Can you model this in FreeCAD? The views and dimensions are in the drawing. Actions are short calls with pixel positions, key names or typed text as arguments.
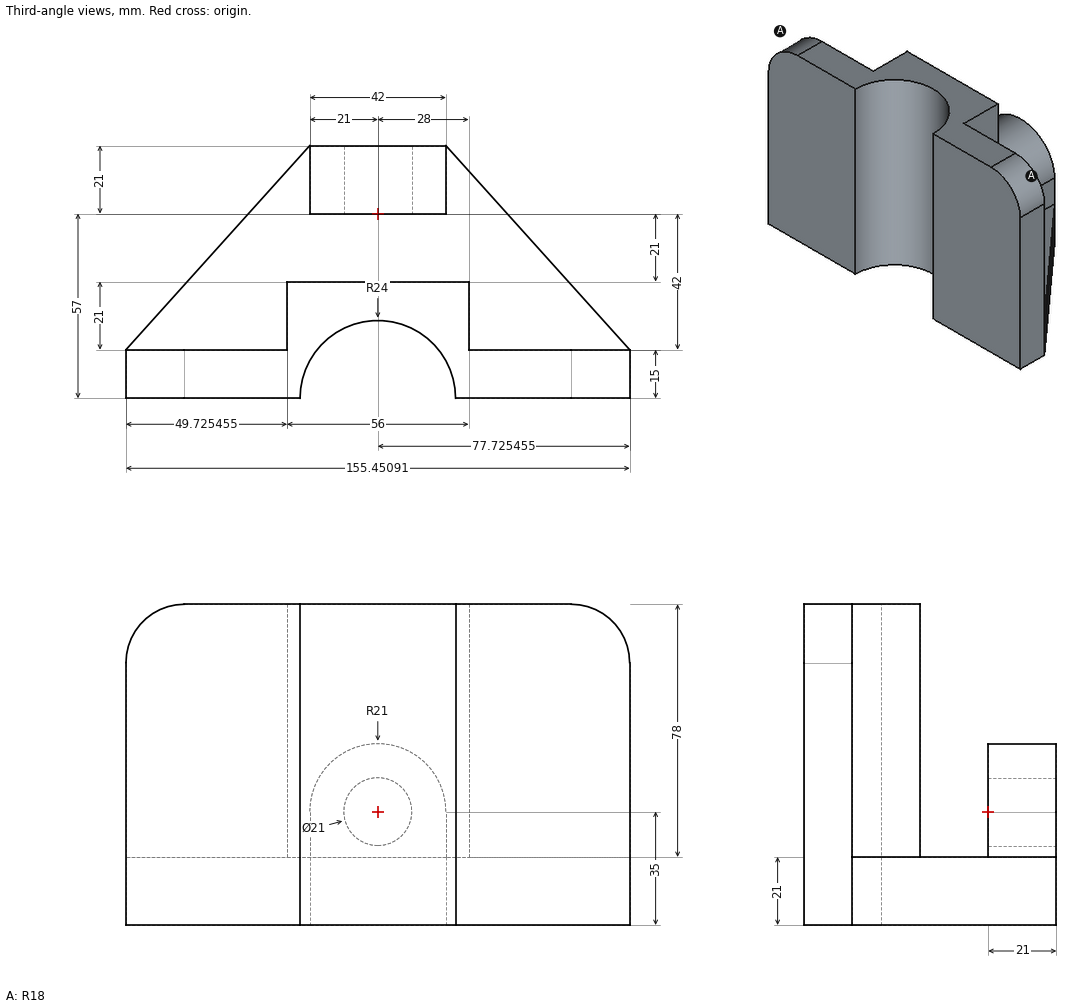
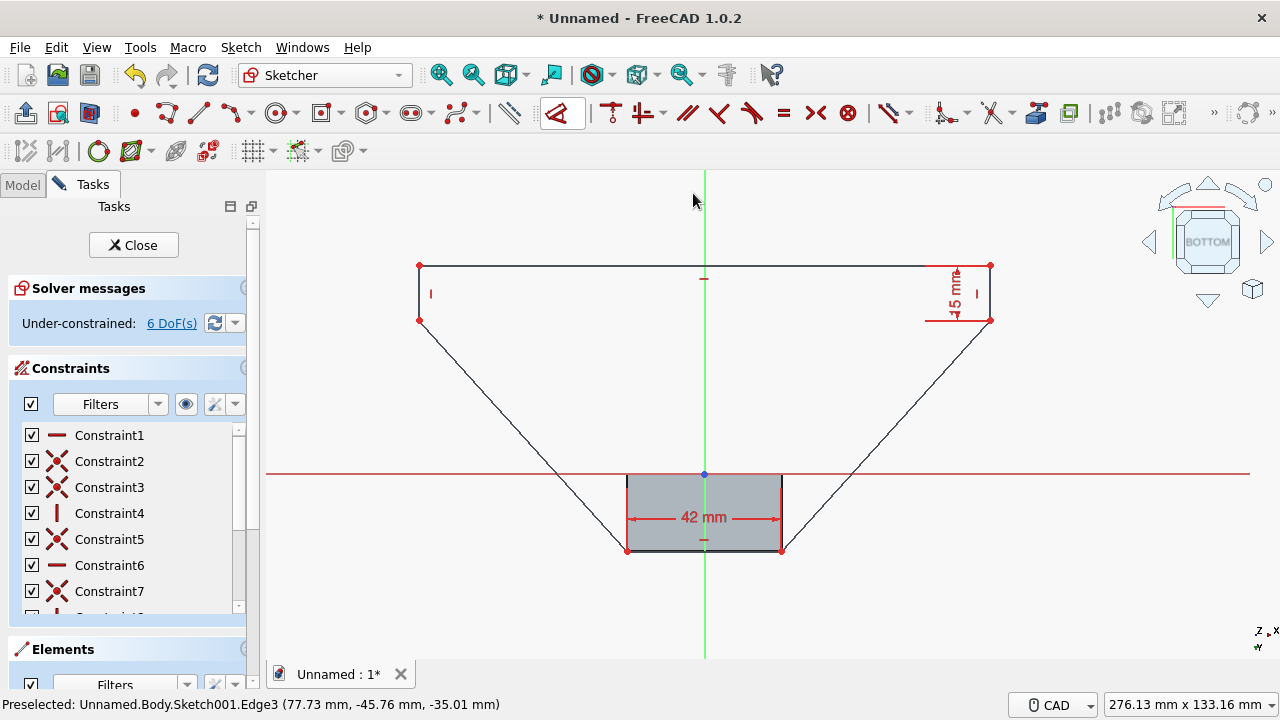
click(419, 282)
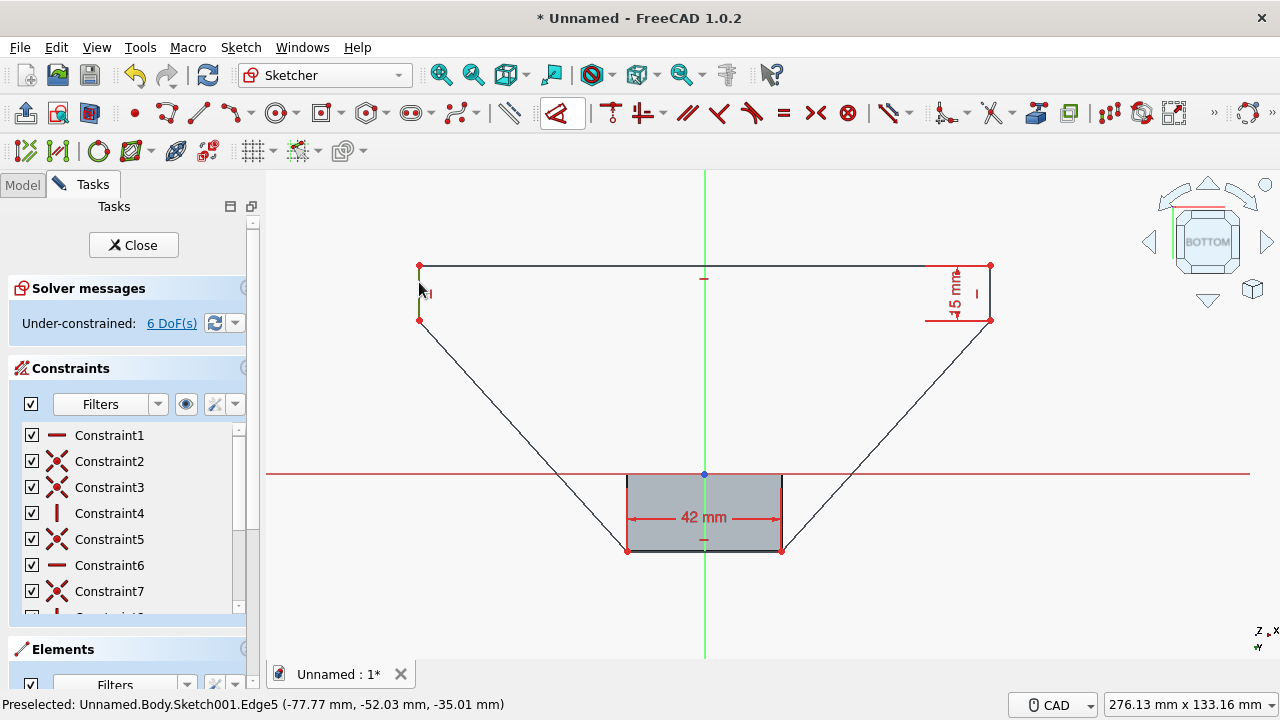
key(i)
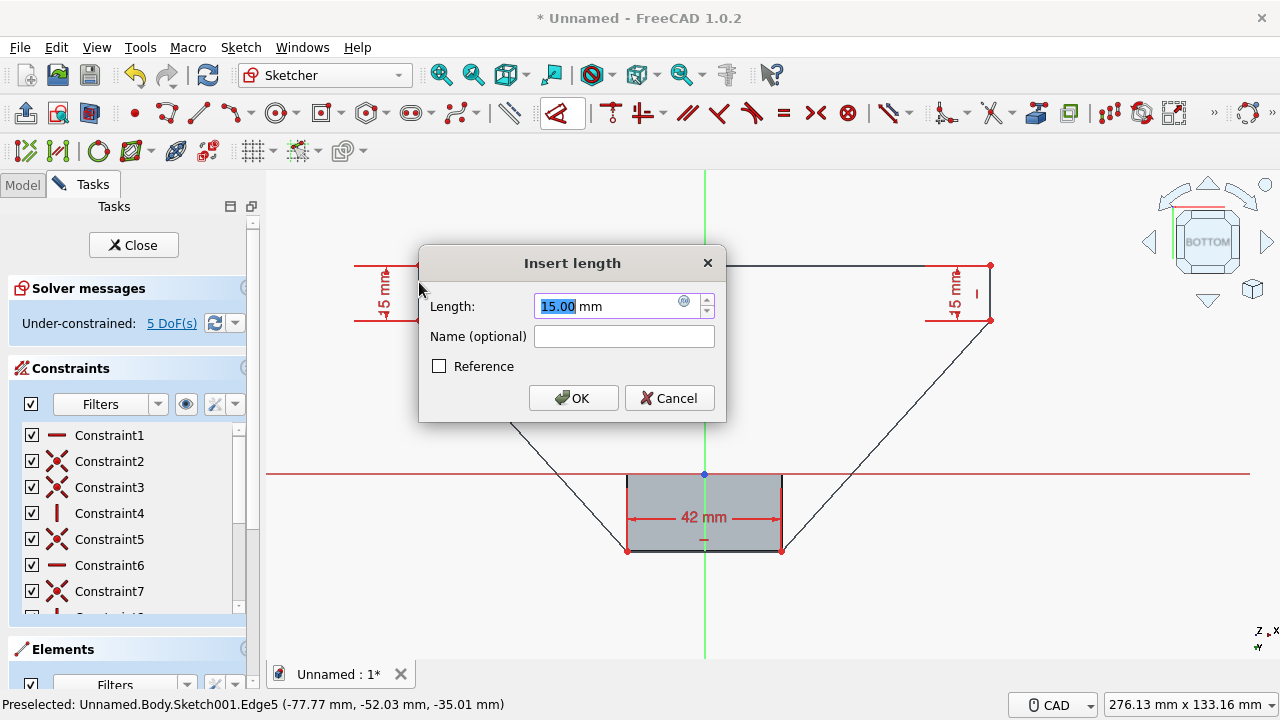
text(15)
key(Return)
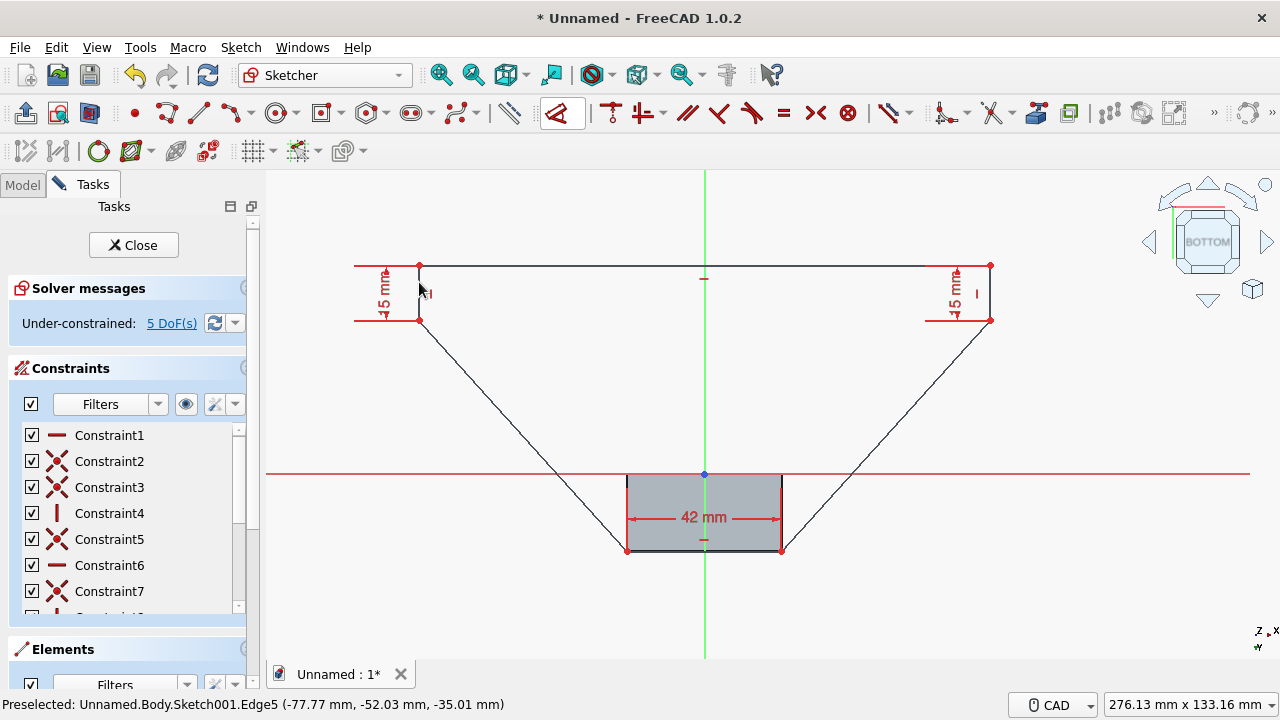
click(627, 552)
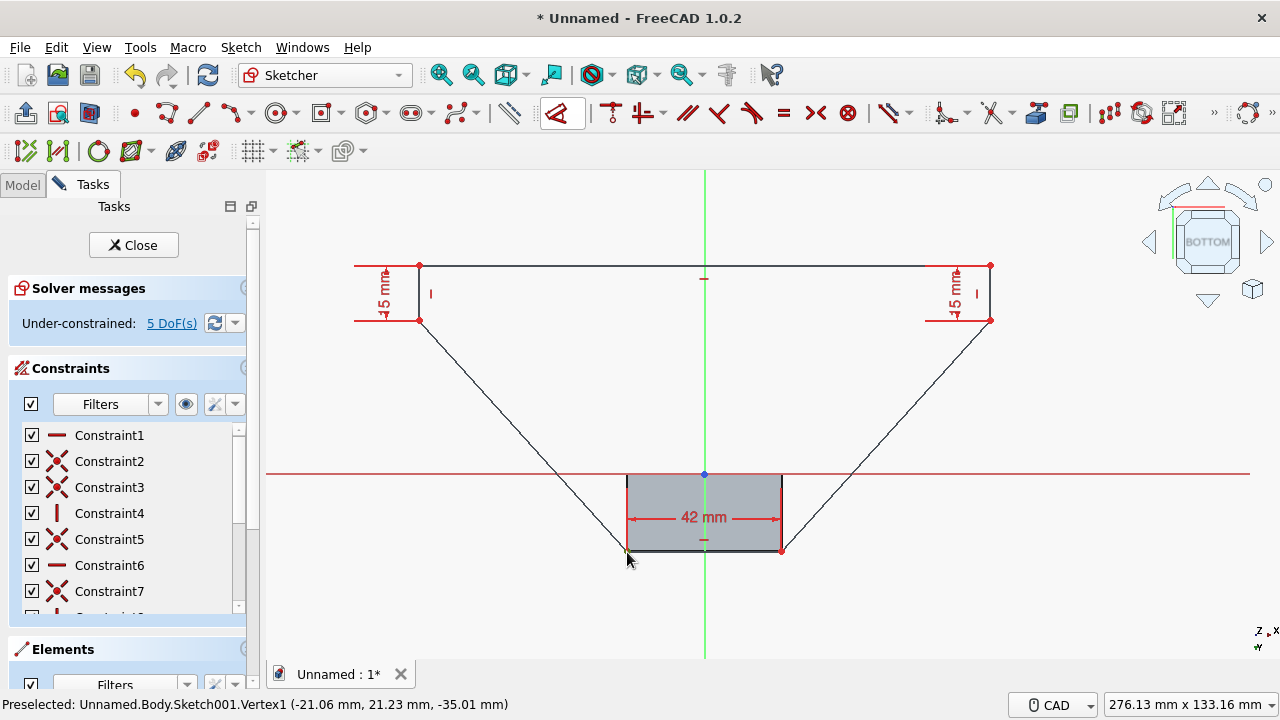
click(580, 114)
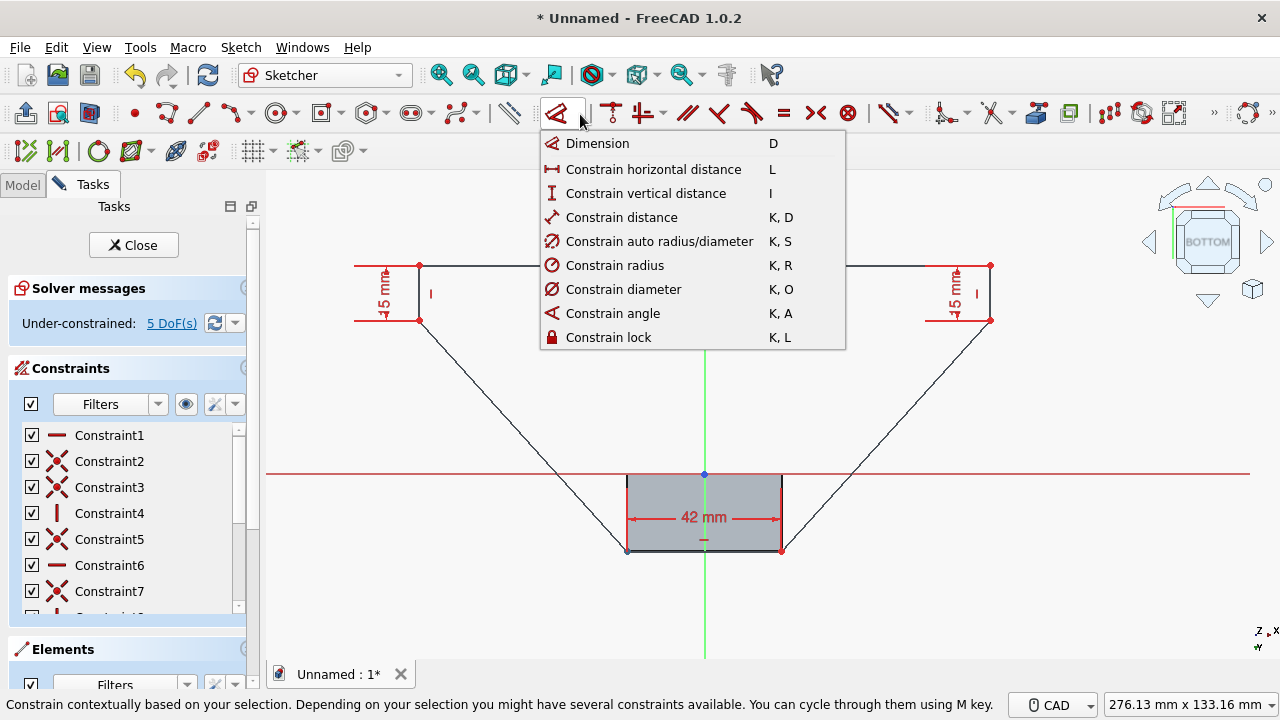
click(693, 169)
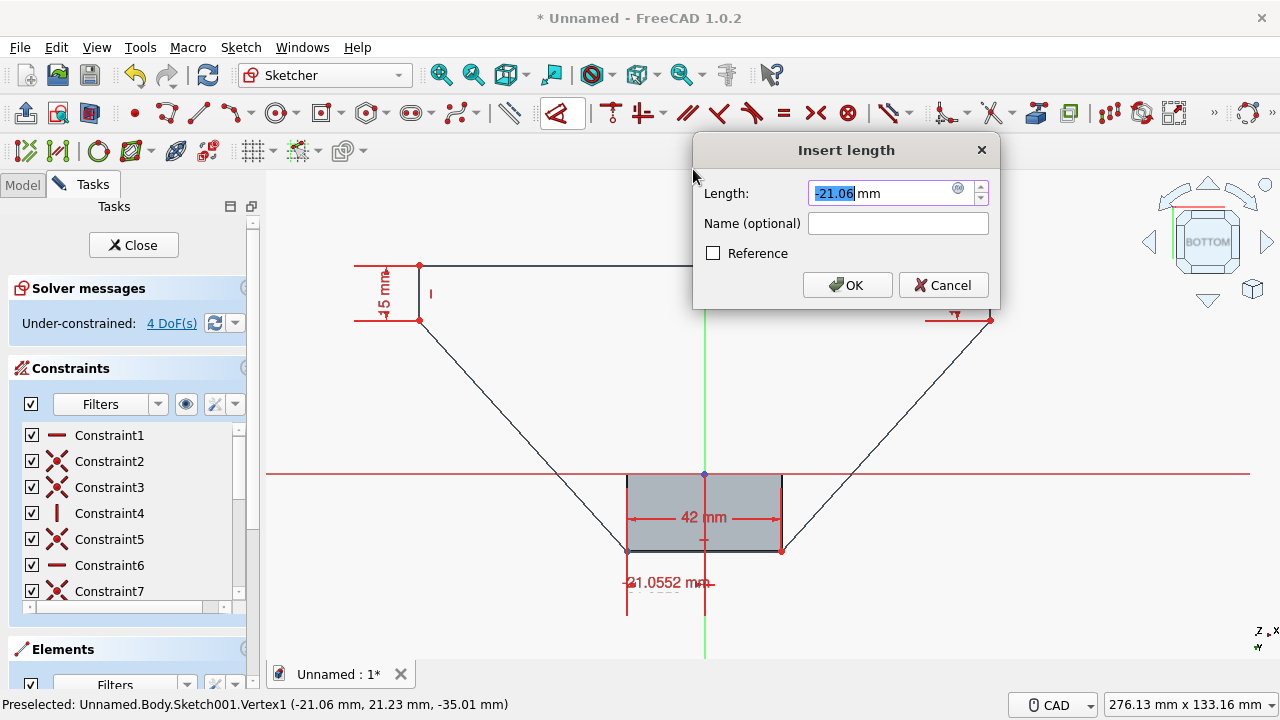
text(-21)
key(Return)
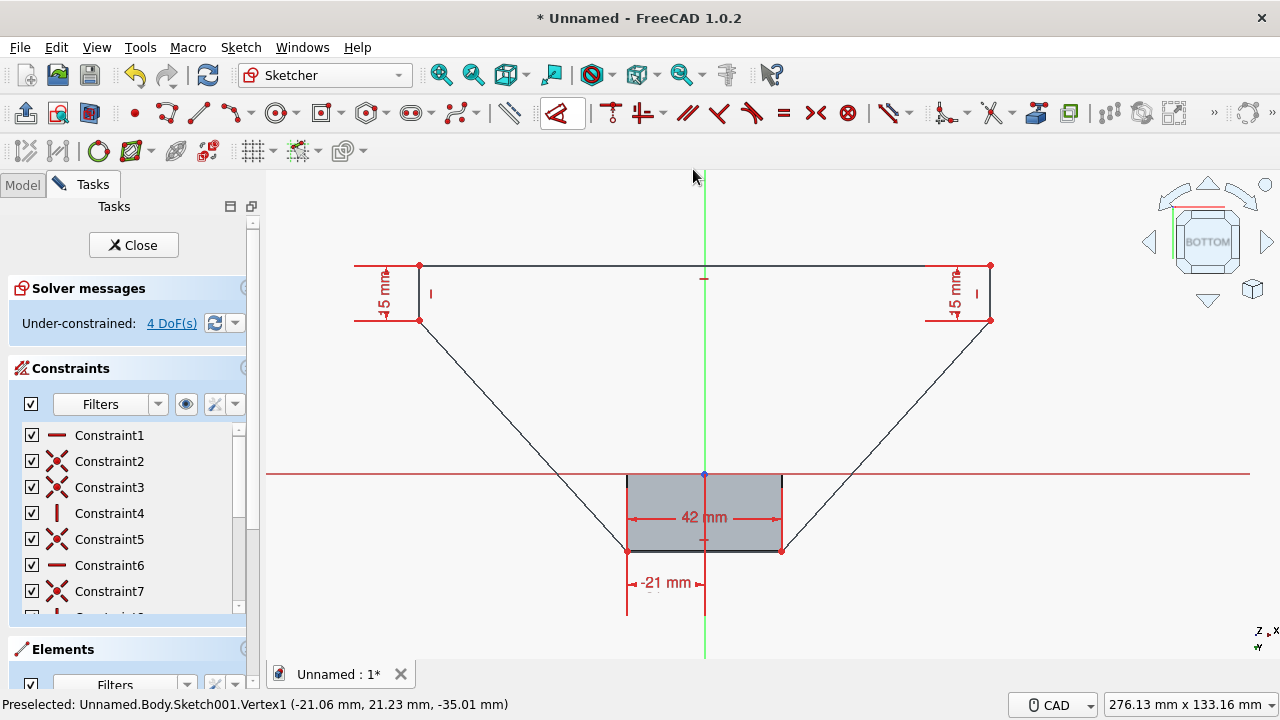
click(627, 552)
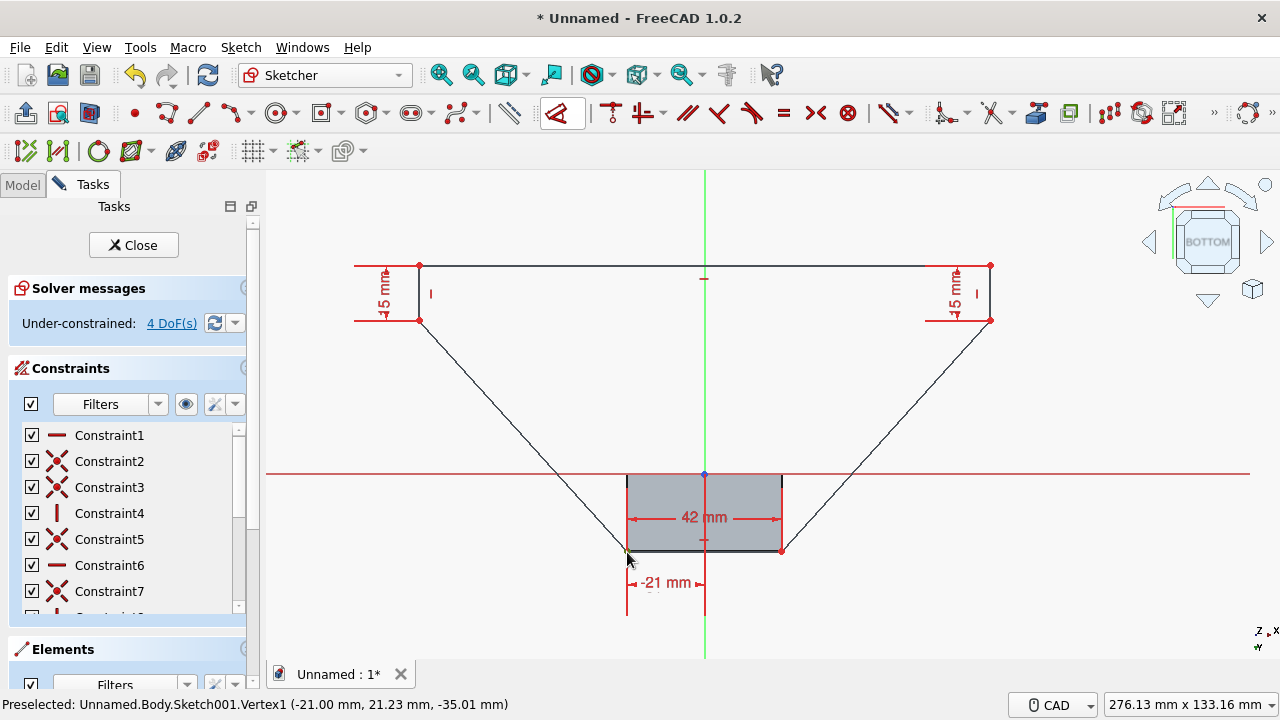
key(i)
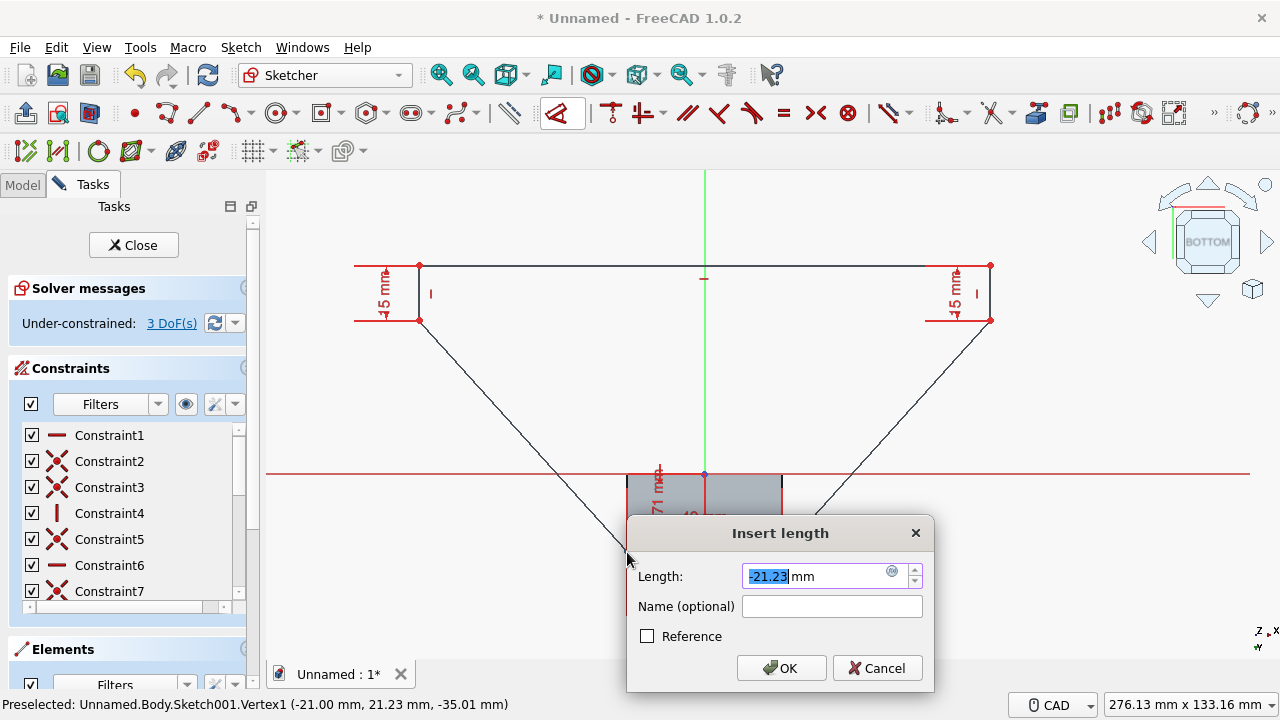
text(-21)
key(Return)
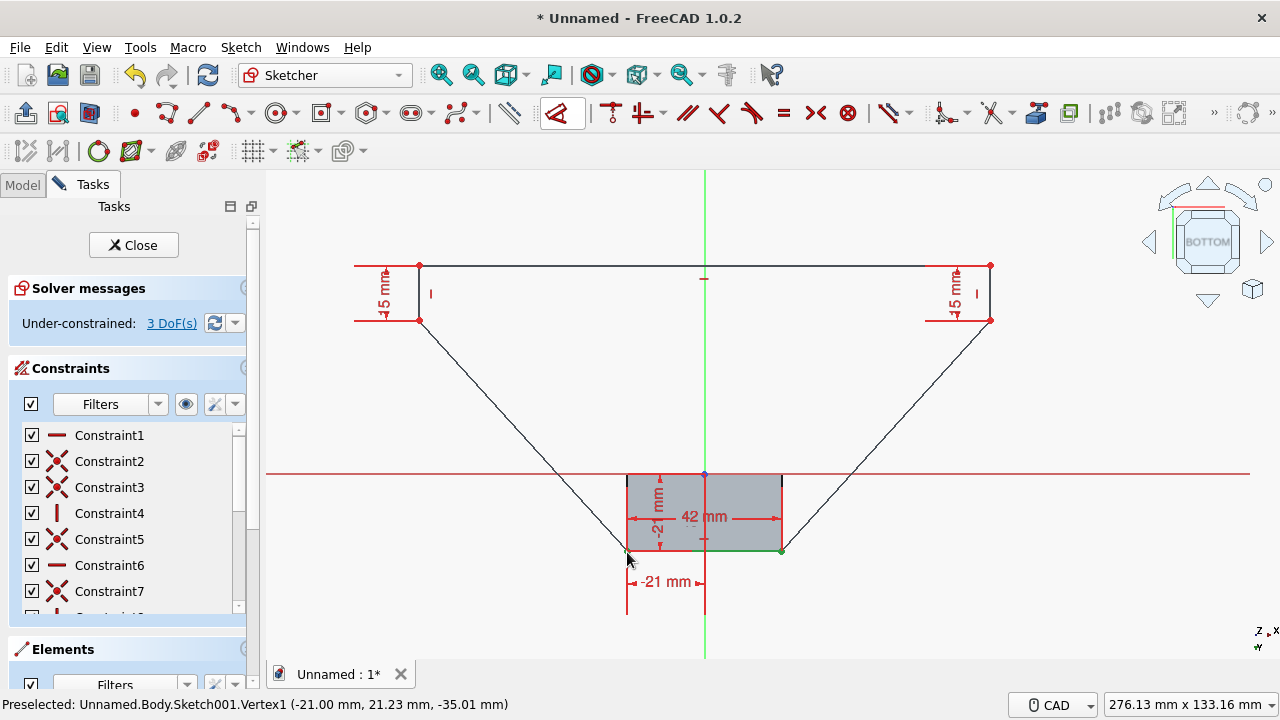
click(990, 321)